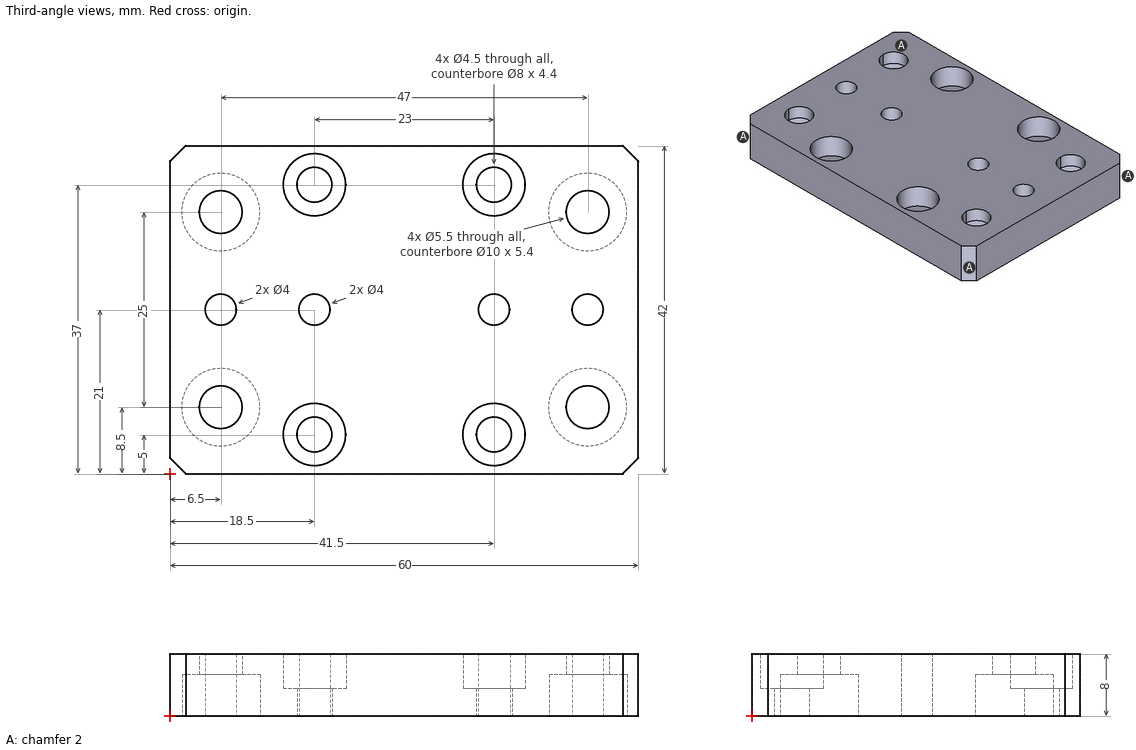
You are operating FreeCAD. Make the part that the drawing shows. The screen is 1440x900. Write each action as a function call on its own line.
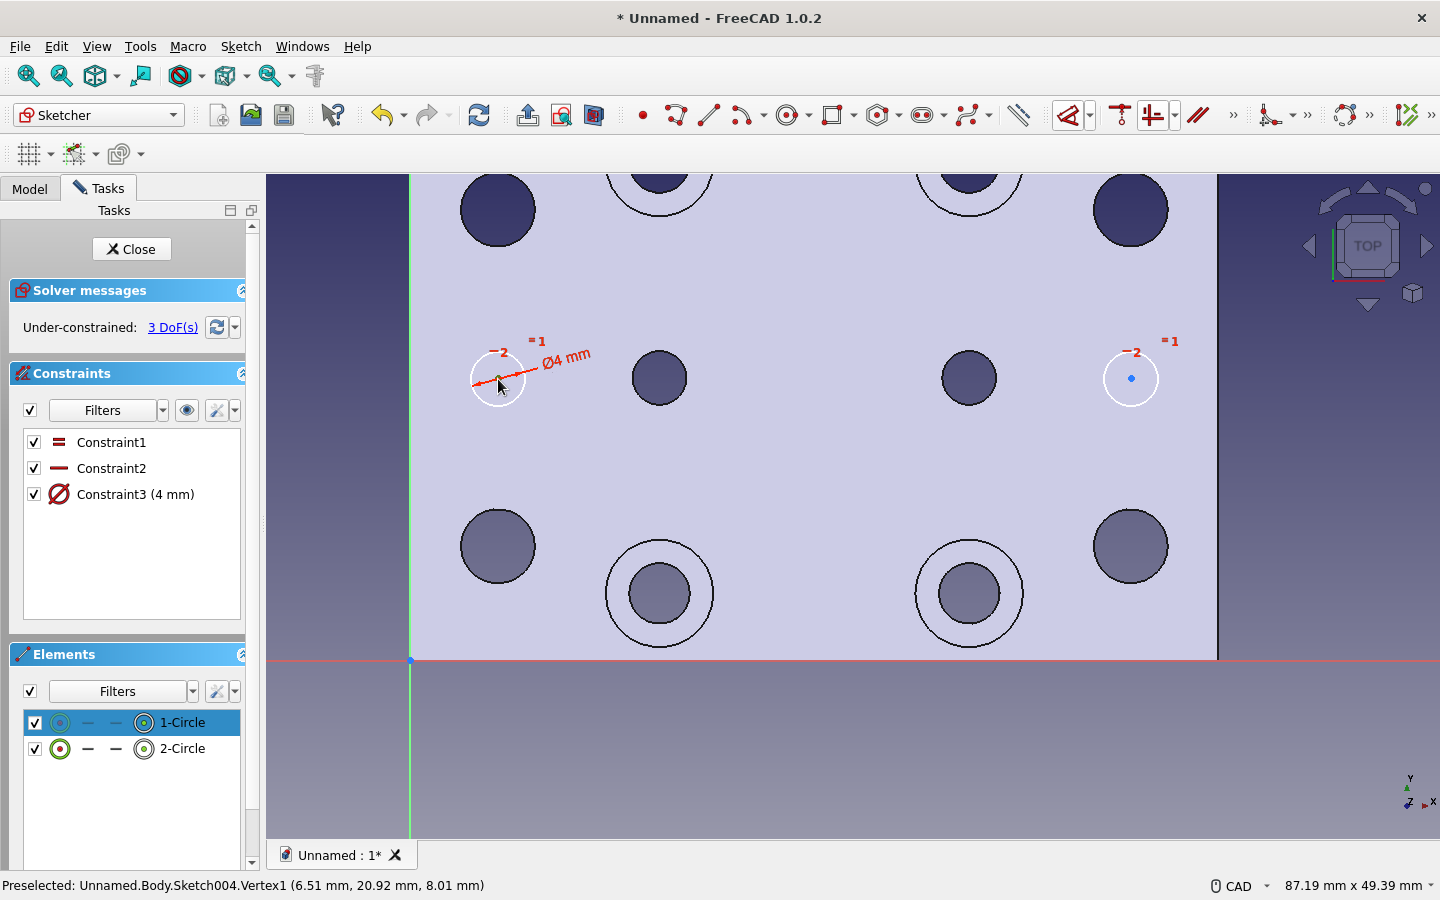
key(i)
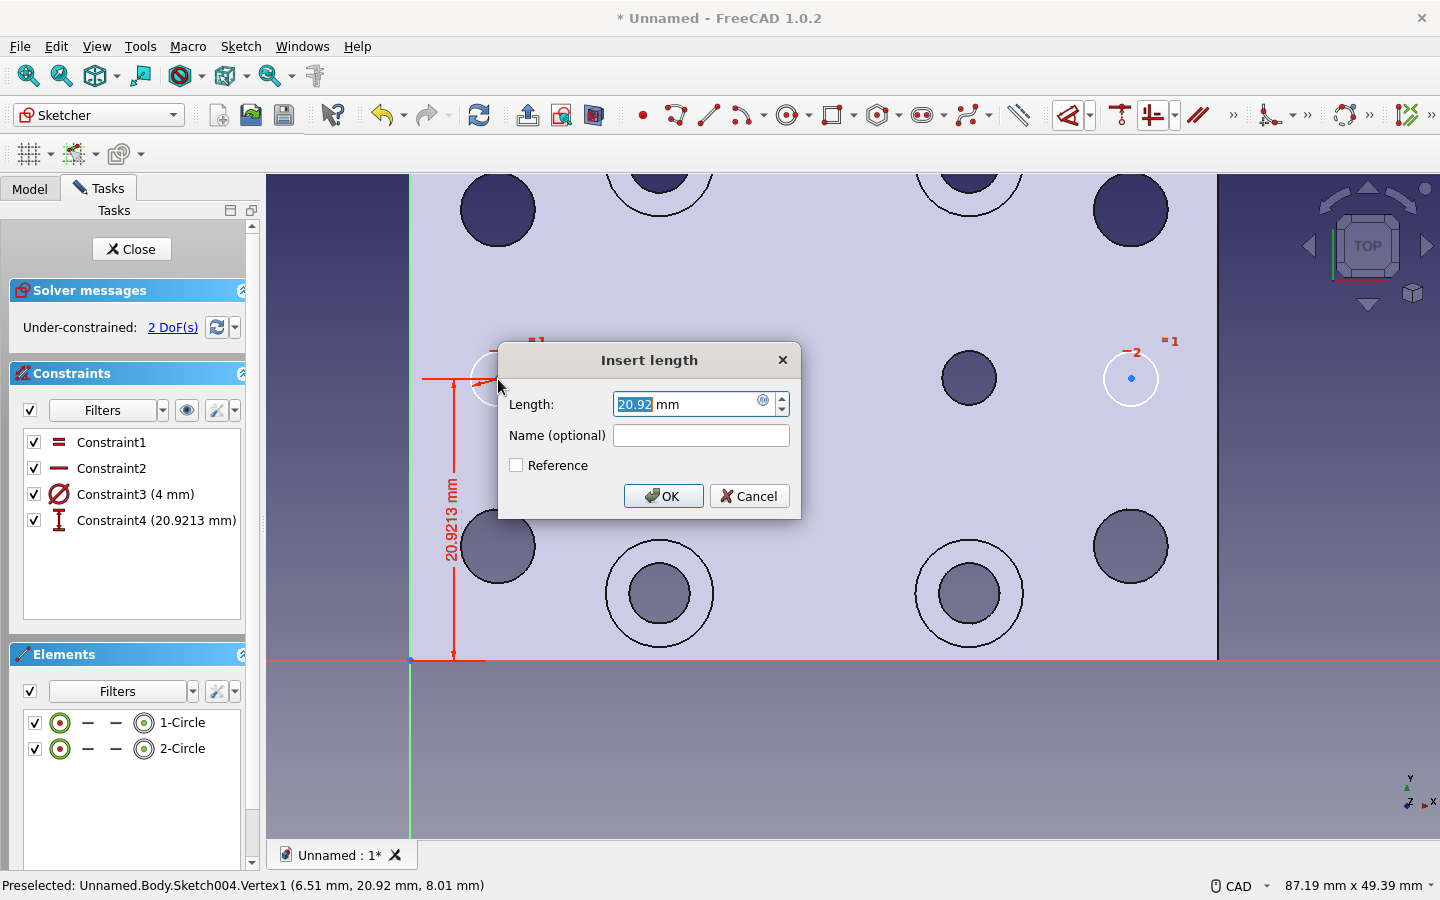
text(21)
key(Return)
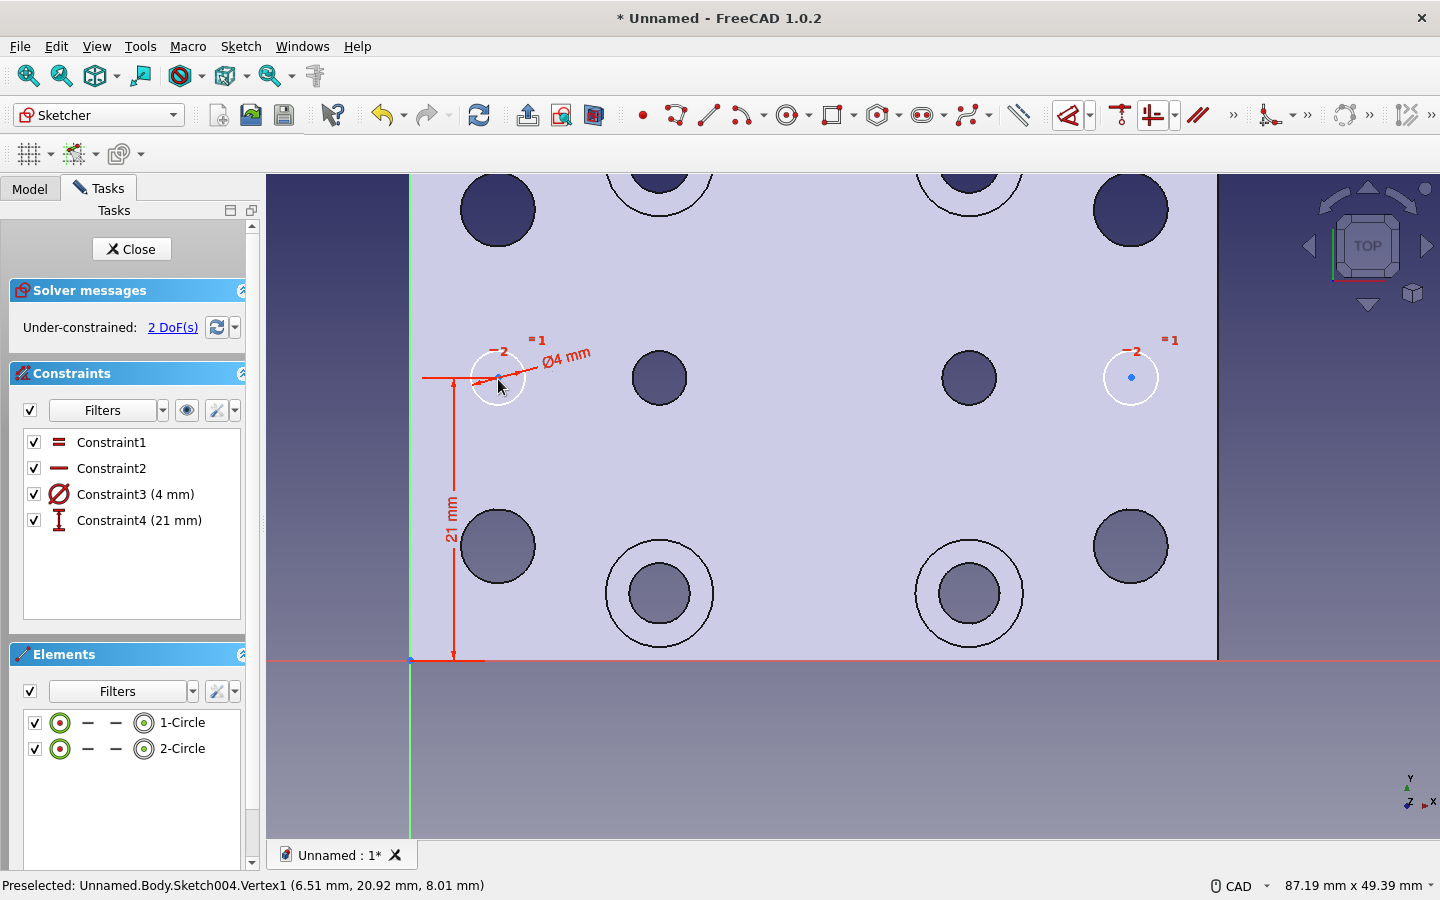
click(498, 378)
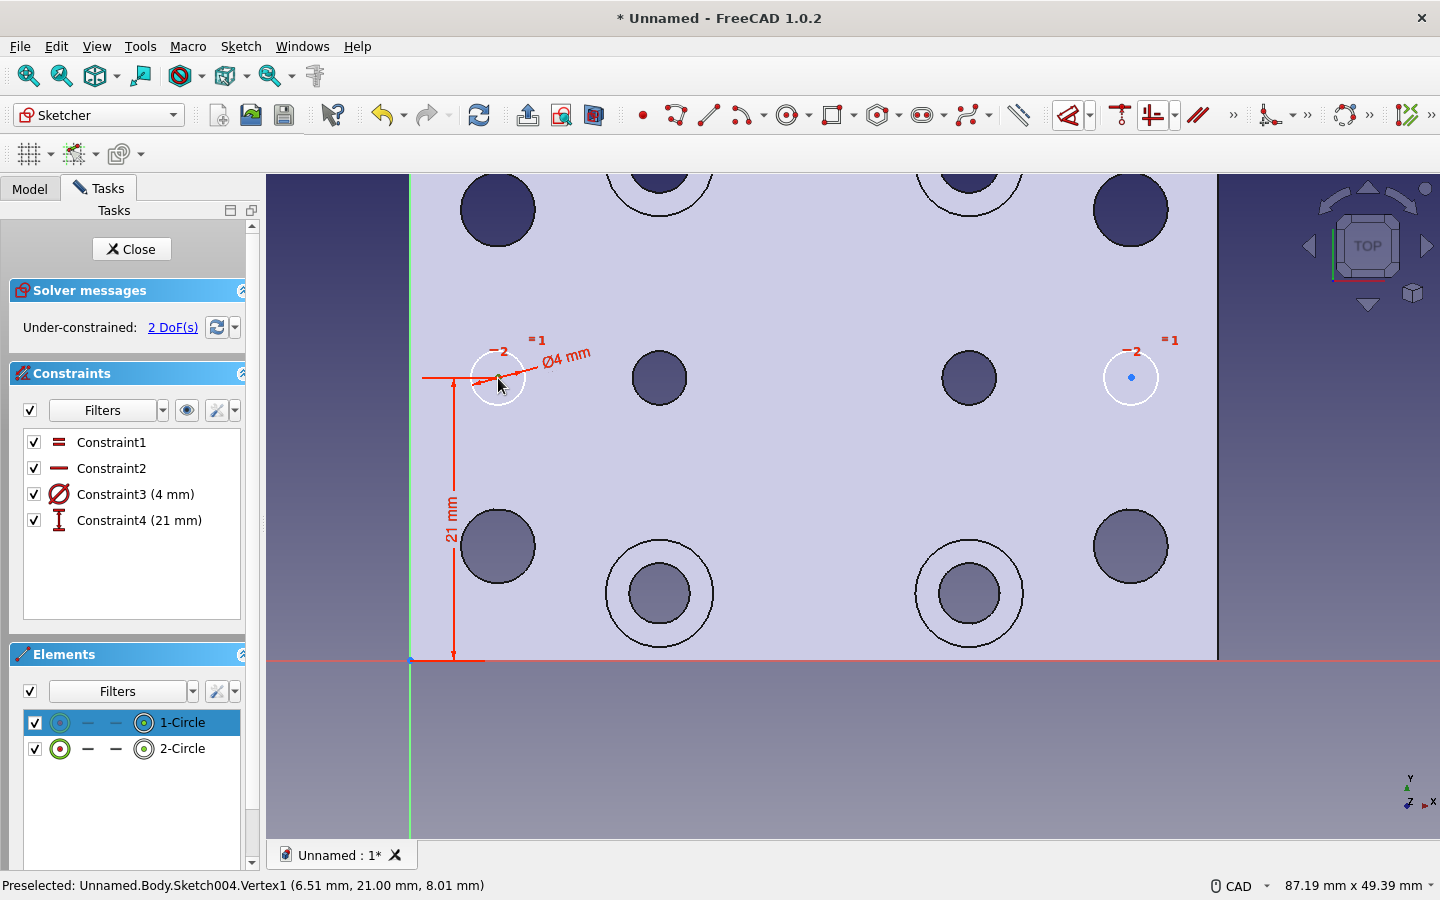
click(1090, 116)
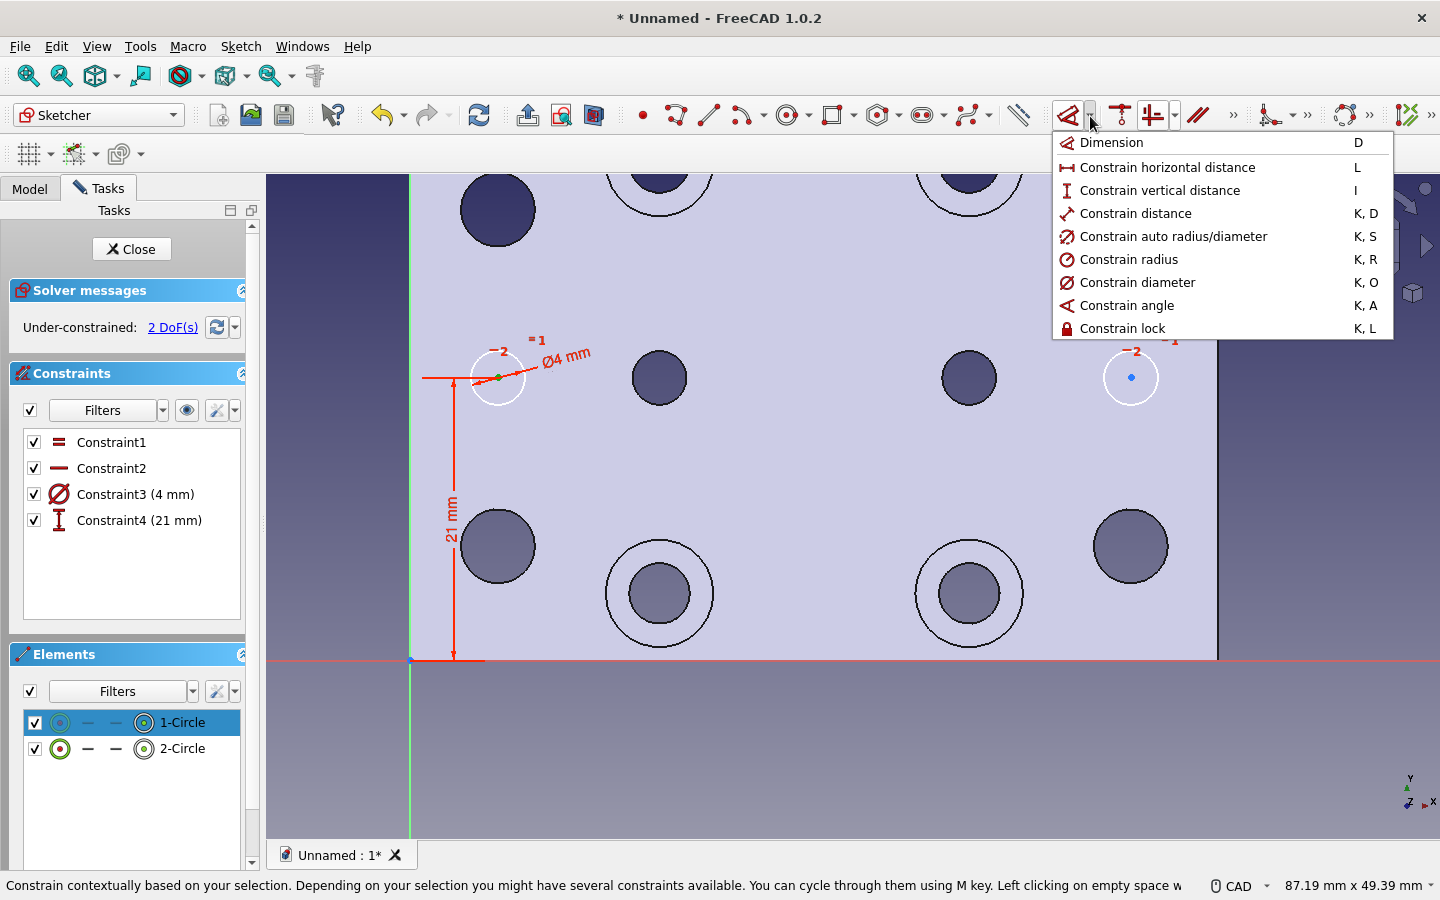
click(1223, 168)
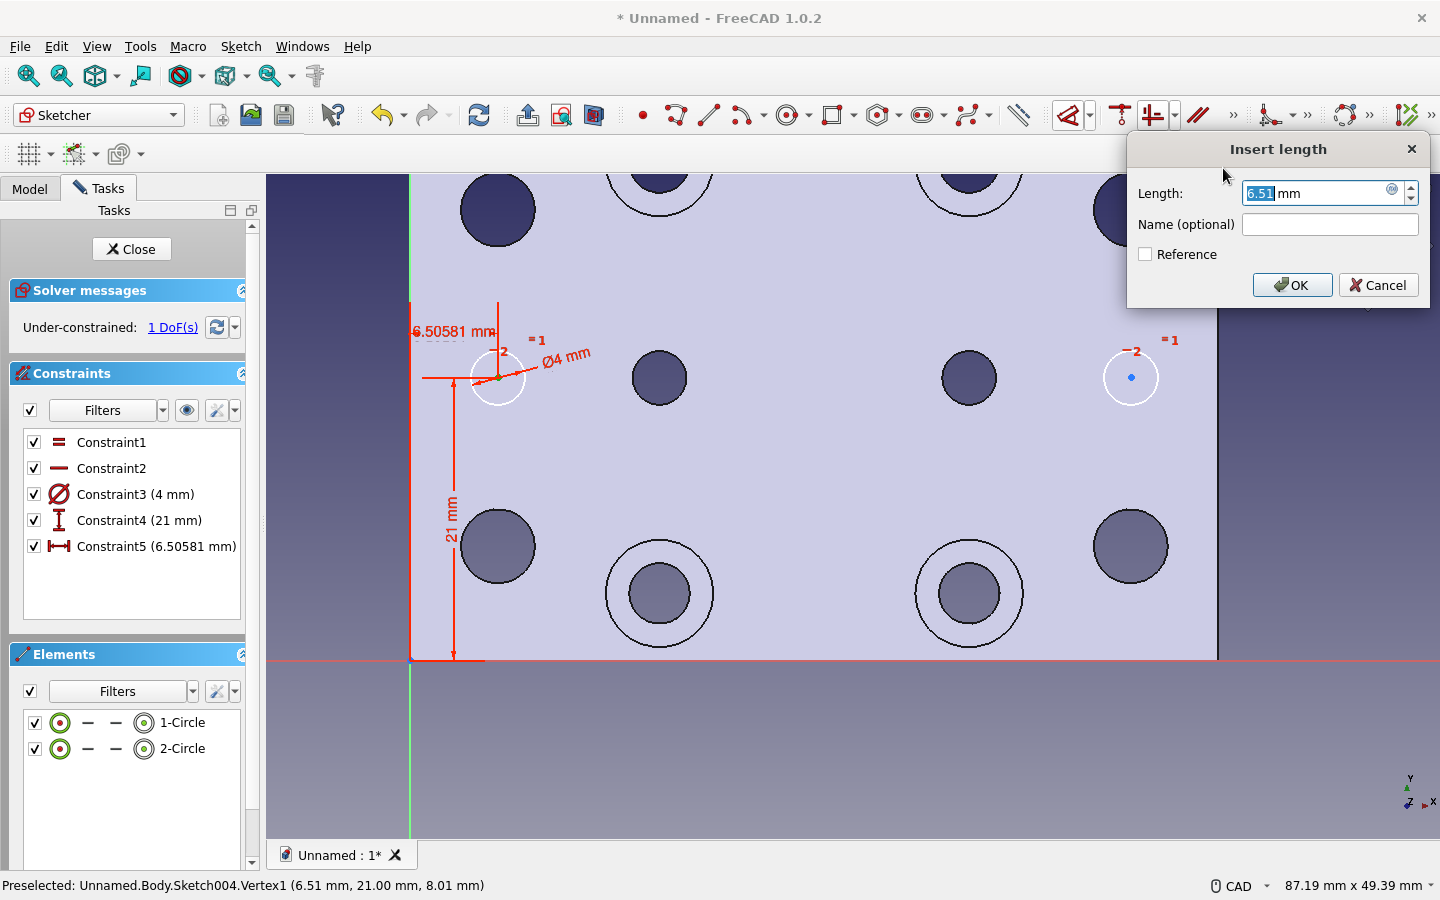
text(6.5)
key(Return)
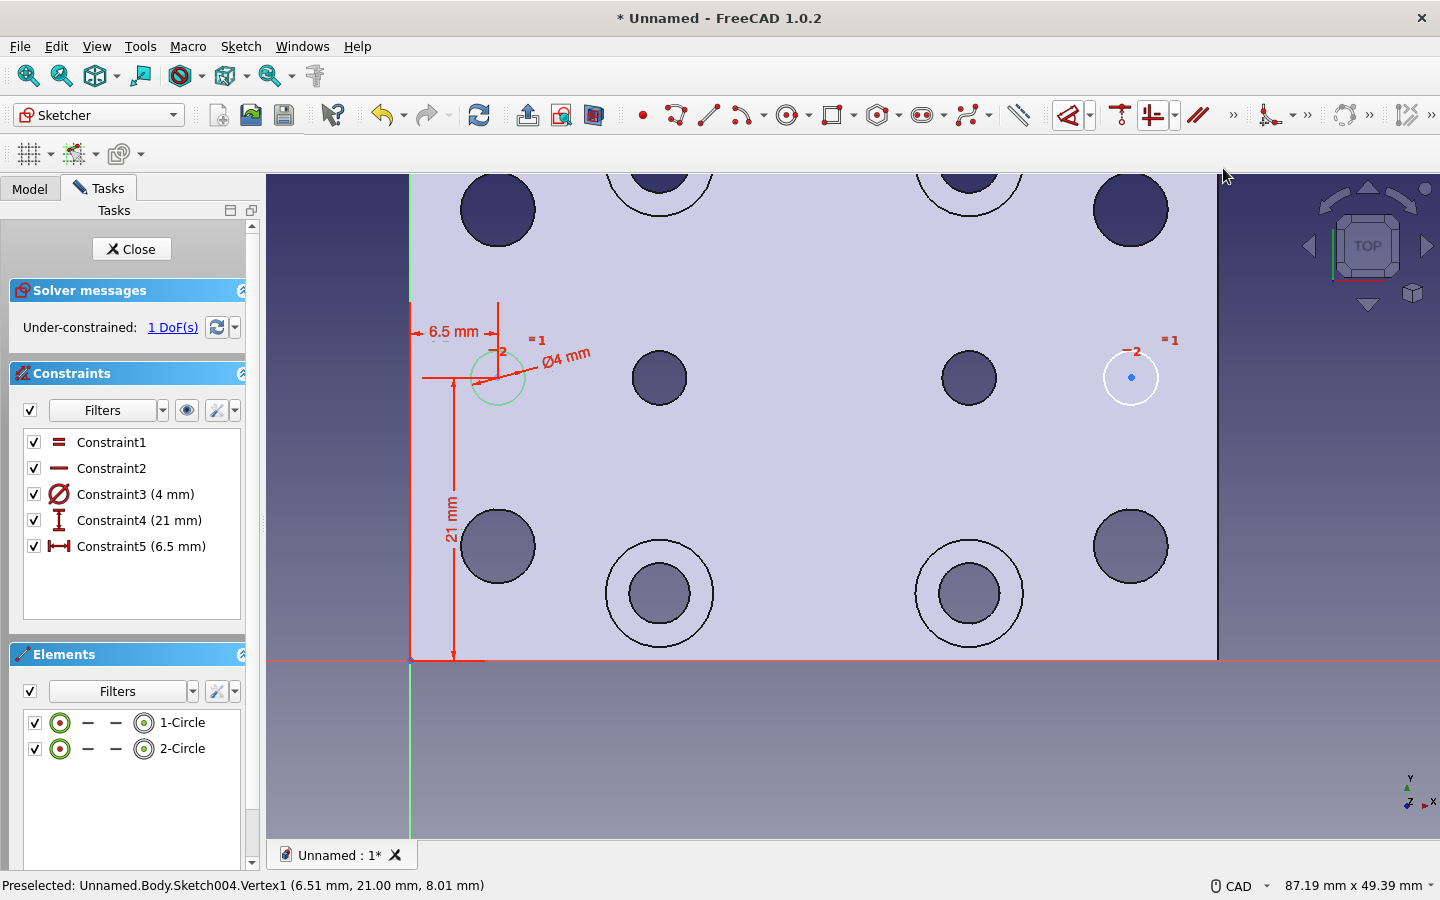
click(498, 378)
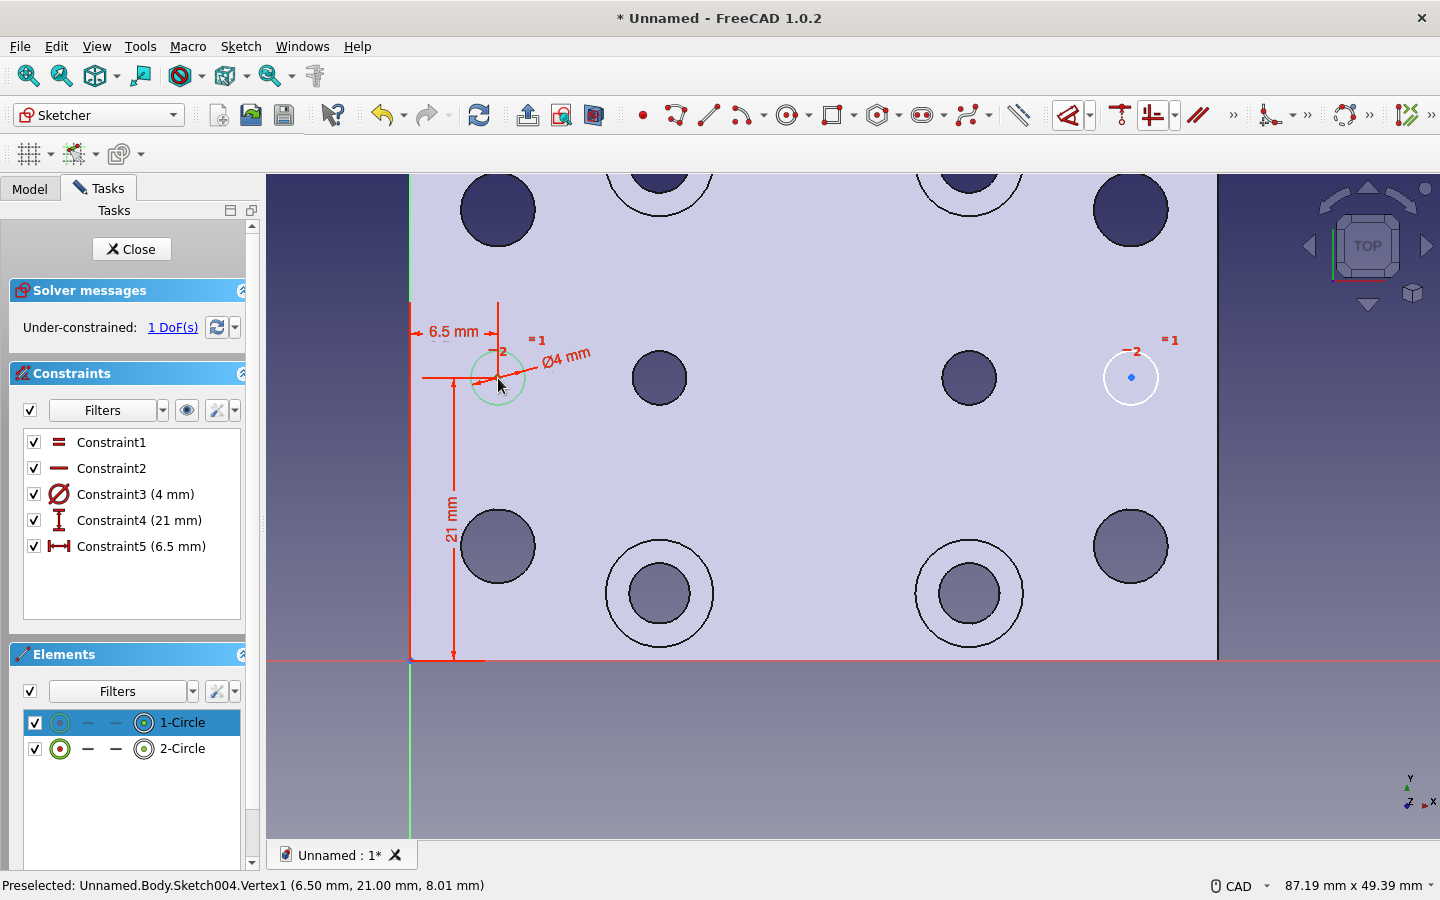
click(1131, 378)